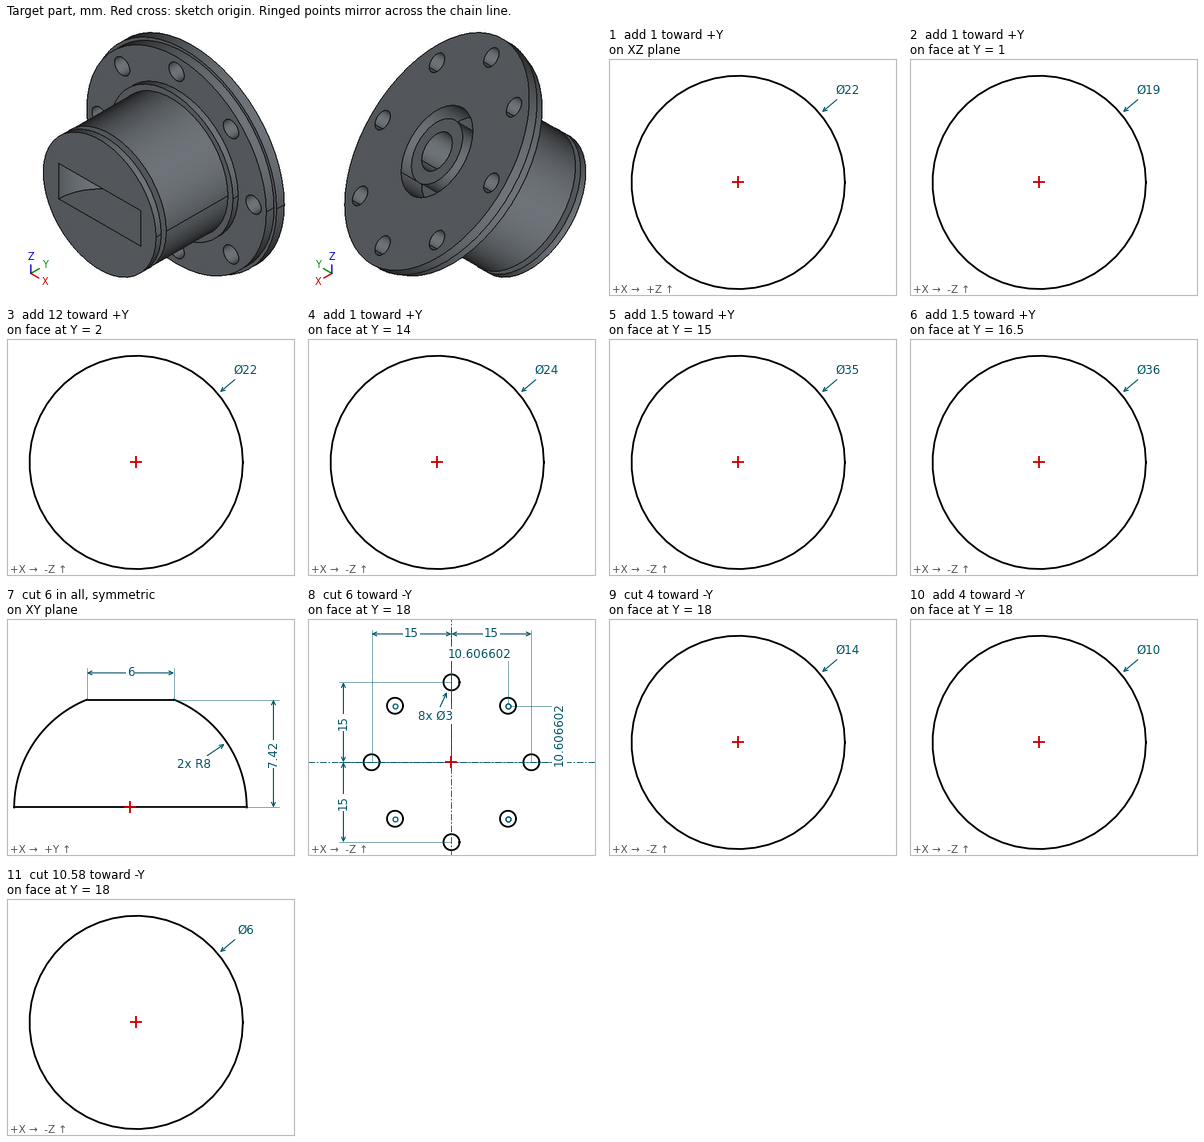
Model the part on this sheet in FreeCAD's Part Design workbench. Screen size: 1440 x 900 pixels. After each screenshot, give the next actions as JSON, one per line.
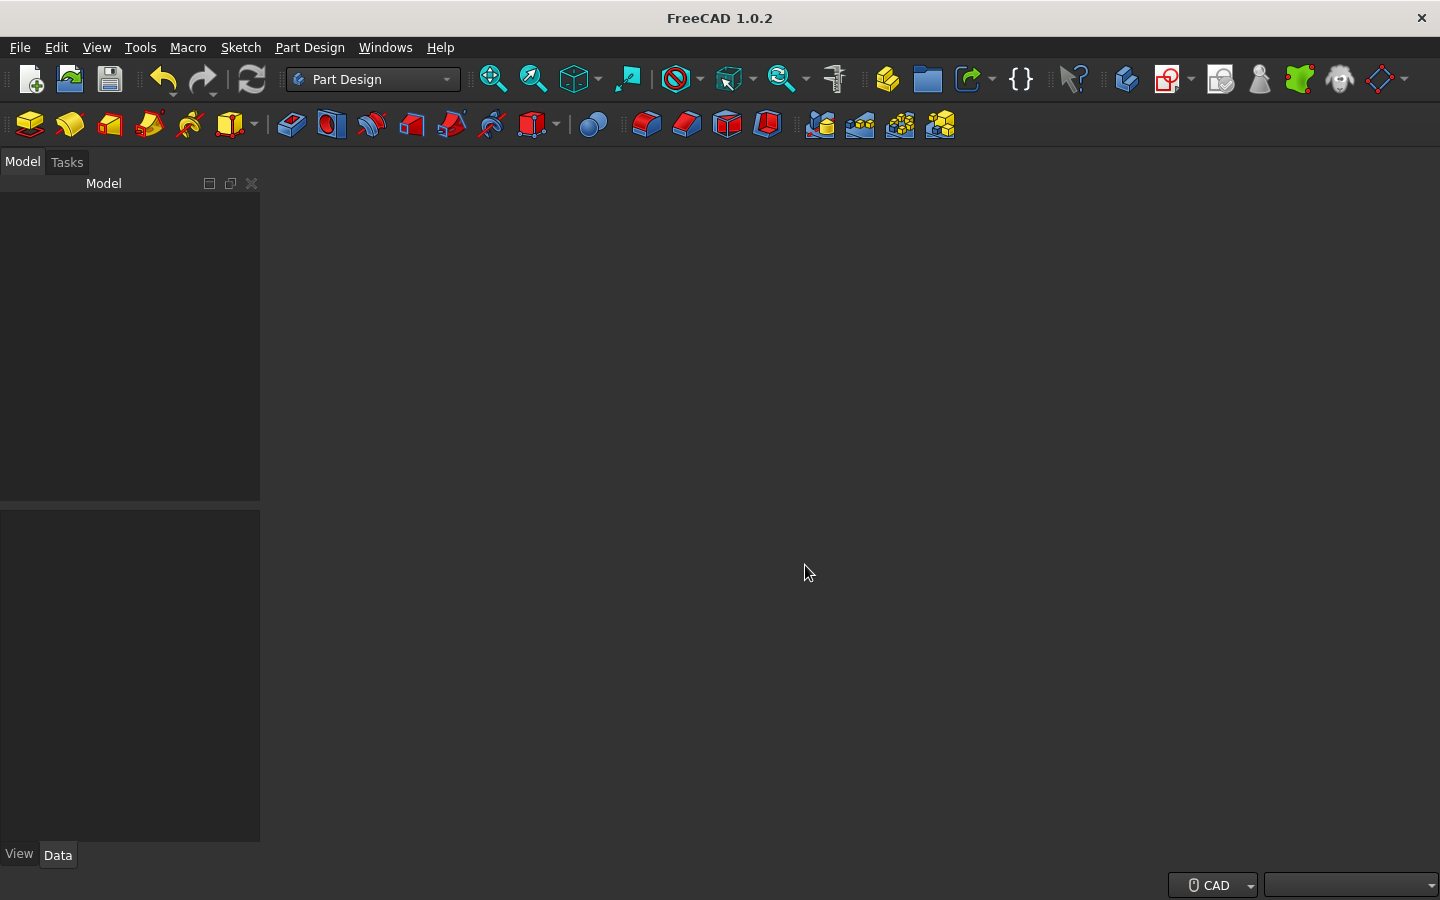
{"action": "left_click", "coordinate": [30, 80]}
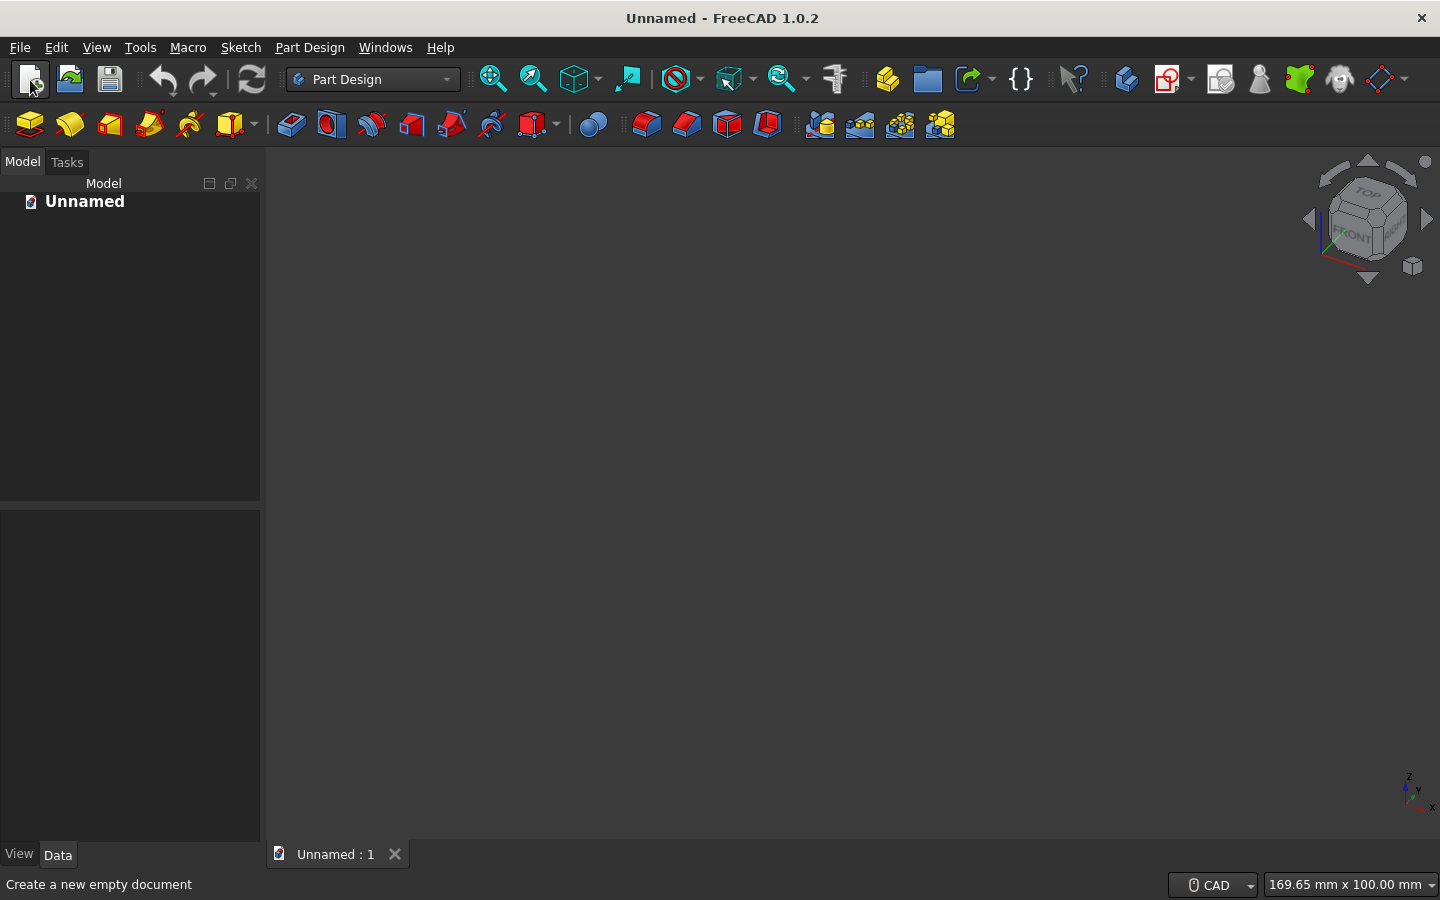
{"action": "left_click", "coordinate": [1168, 80]}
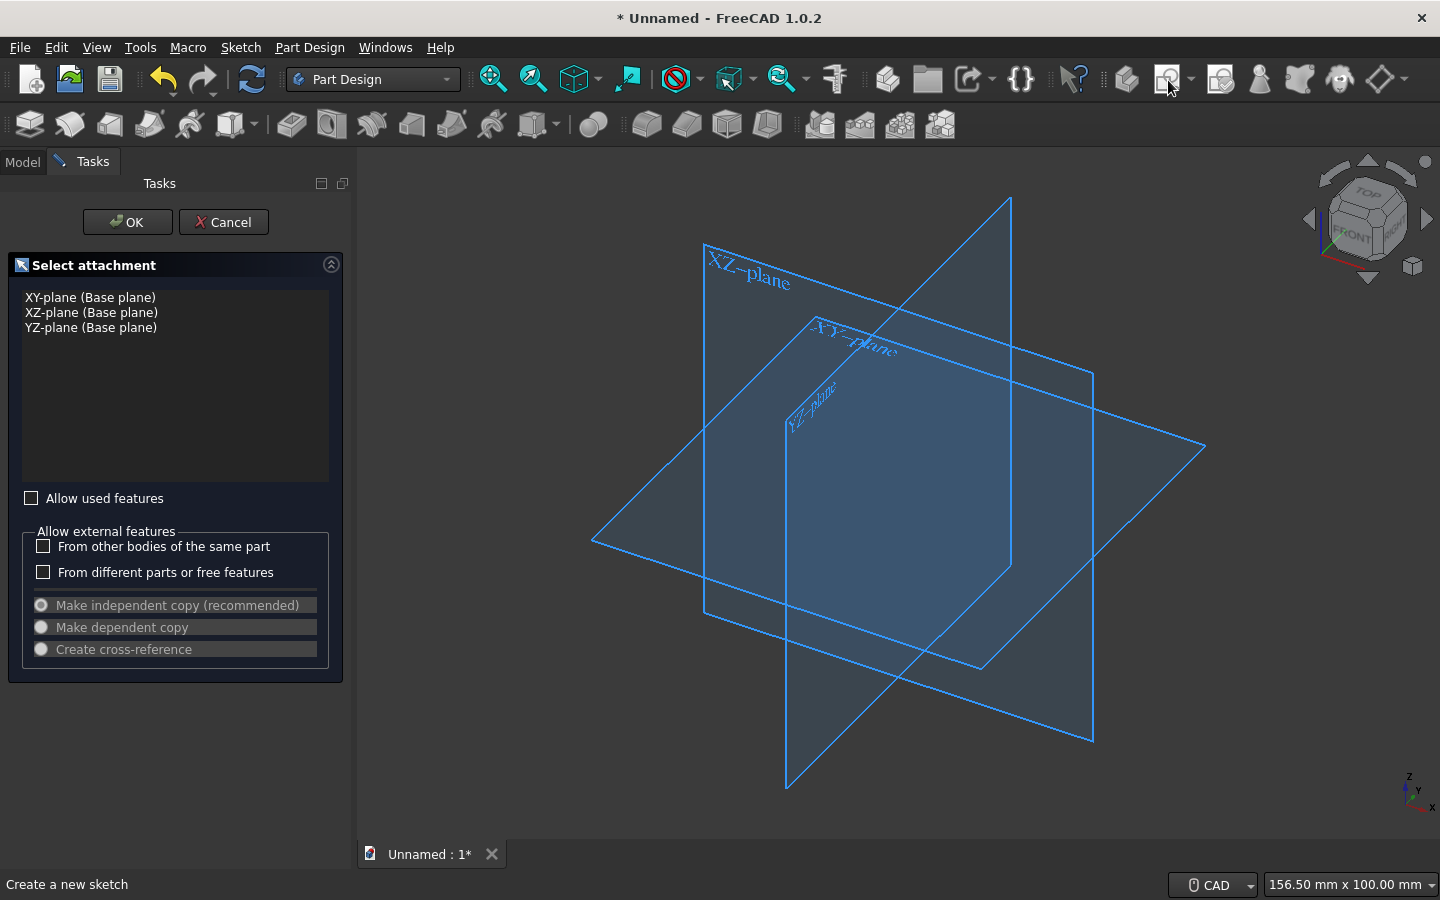
{"action": "left_click", "coordinate": [82, 312]}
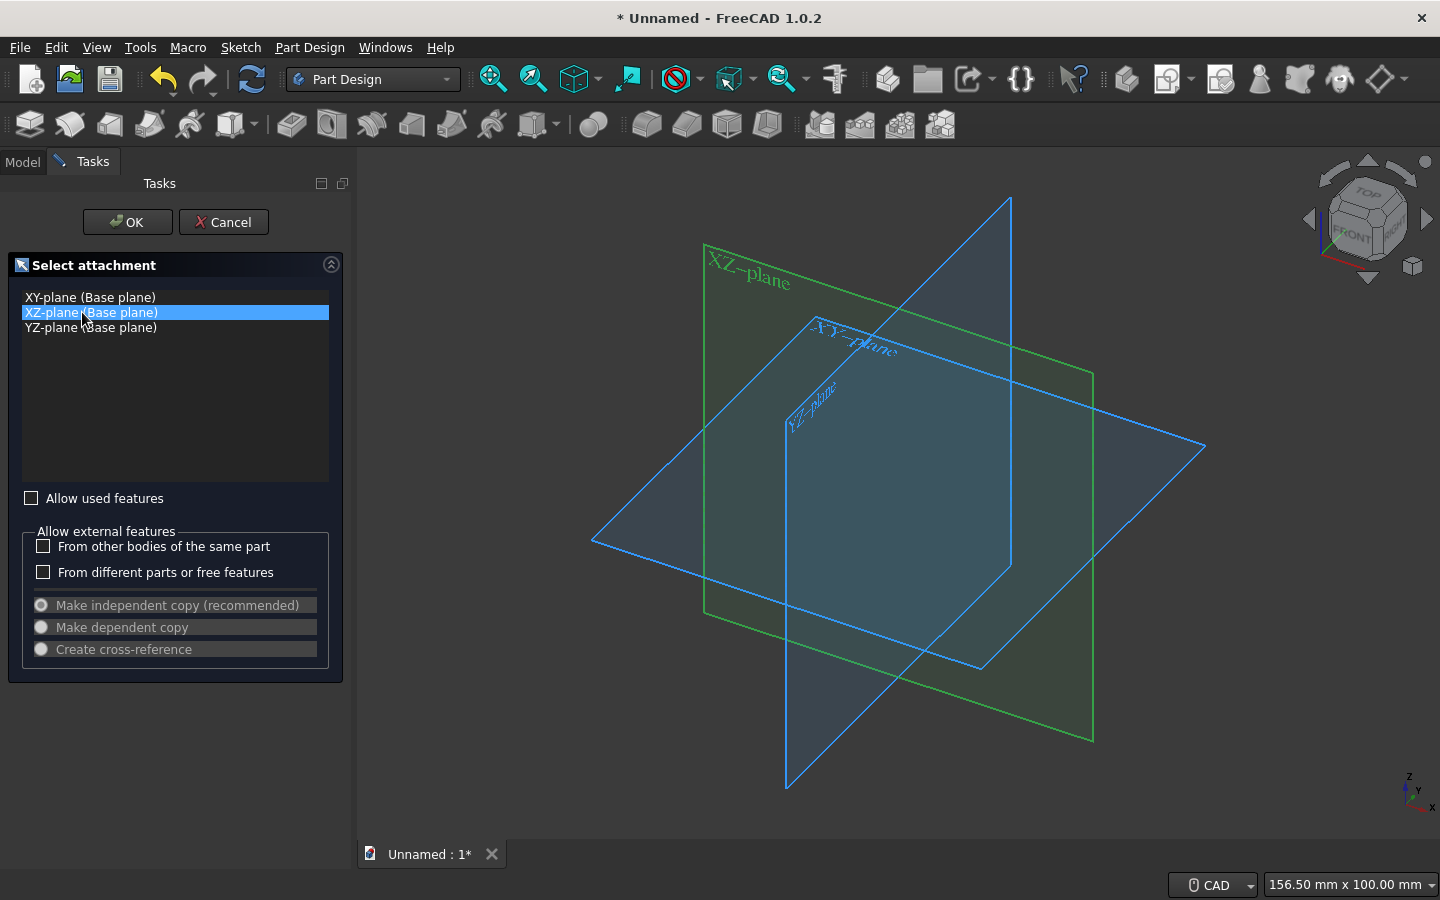
{"action": "left_click", "coordinate": [128, 222]}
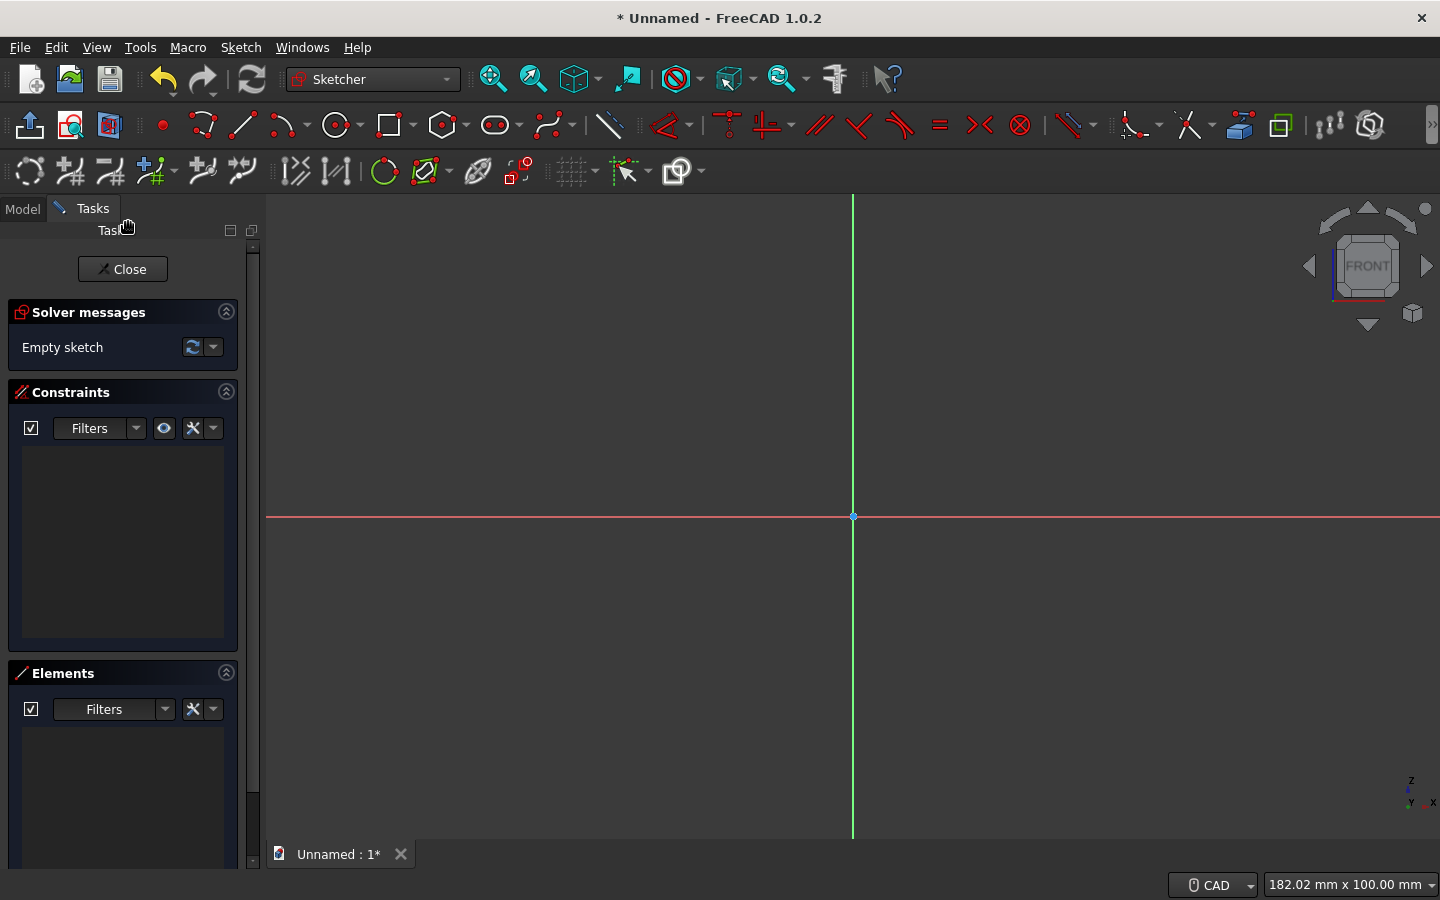
{"action": "scroll", "coordinate": [893, 516], "scroll_direction": "up", "scroll_amount": 5}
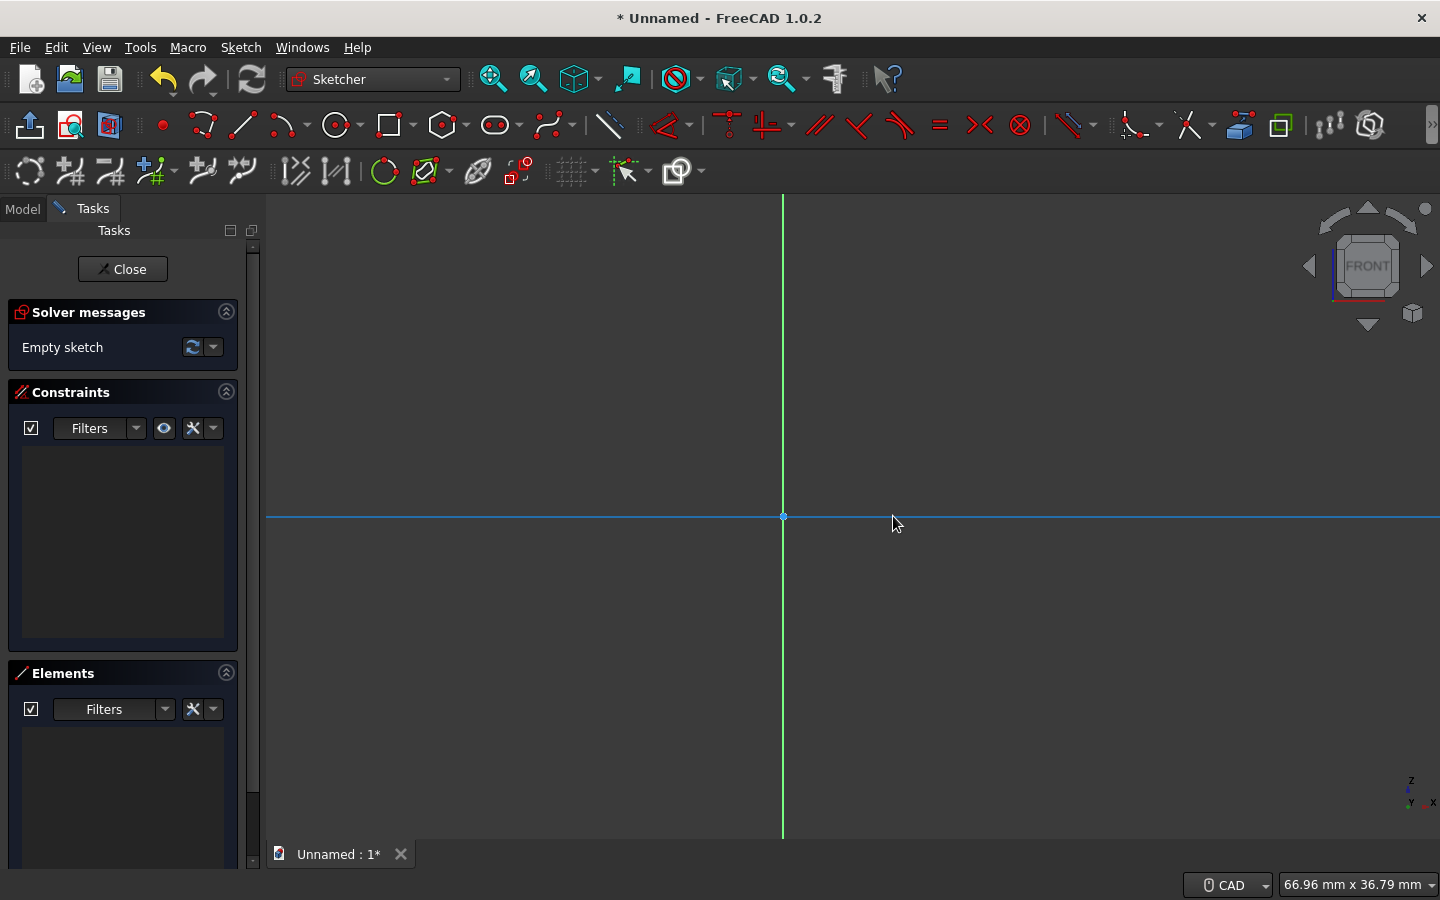
{"action": "left_click", "coordinate": [336, 126]}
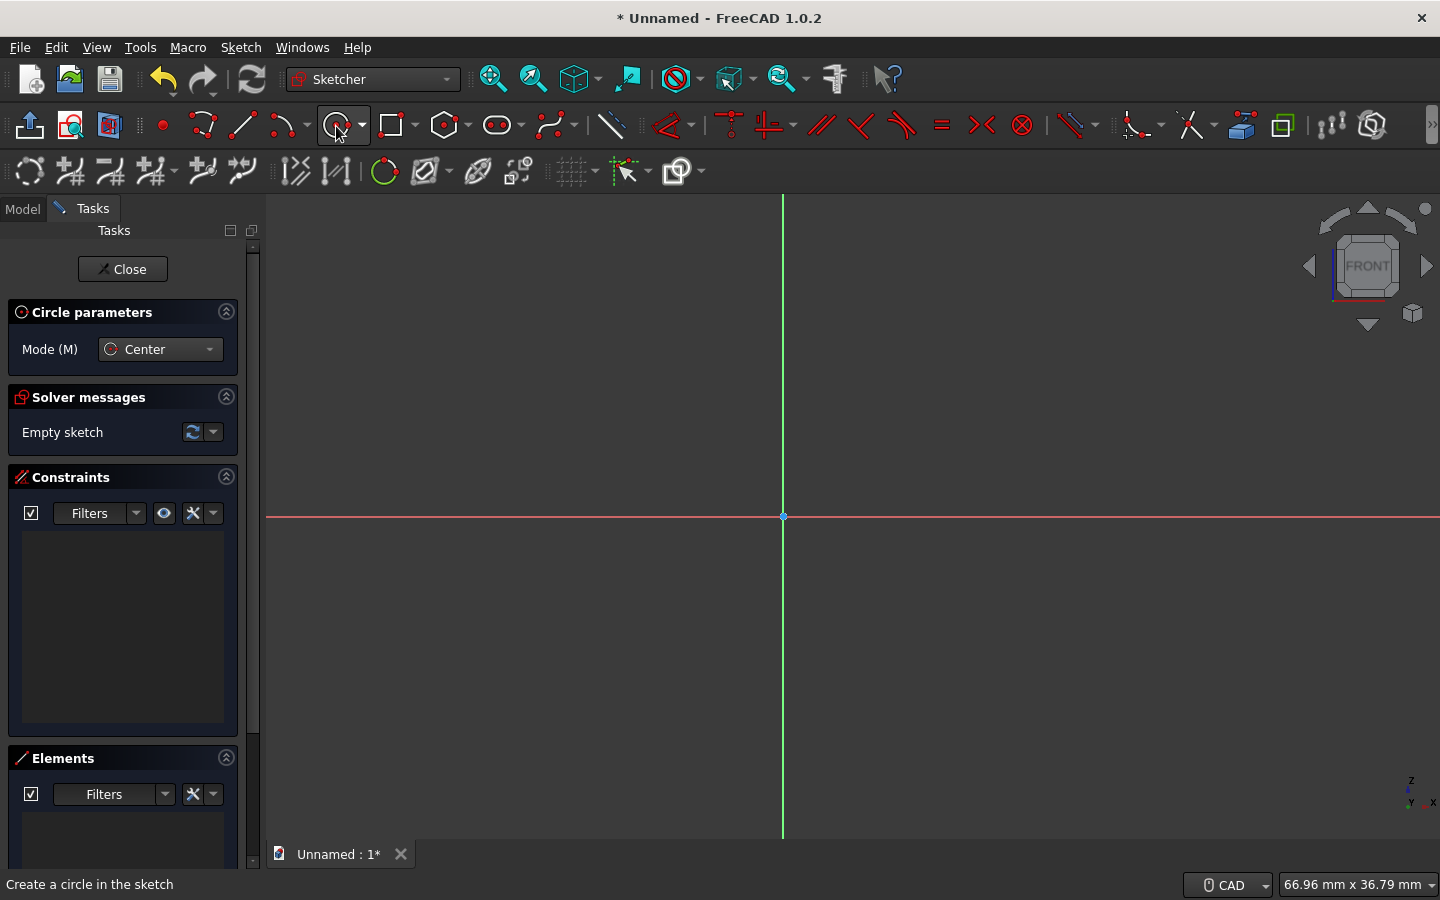
{"action": "left_click", "coordinate": [783, 516]}
{"action": "mouse_move", "coordinate": [920, 380]}